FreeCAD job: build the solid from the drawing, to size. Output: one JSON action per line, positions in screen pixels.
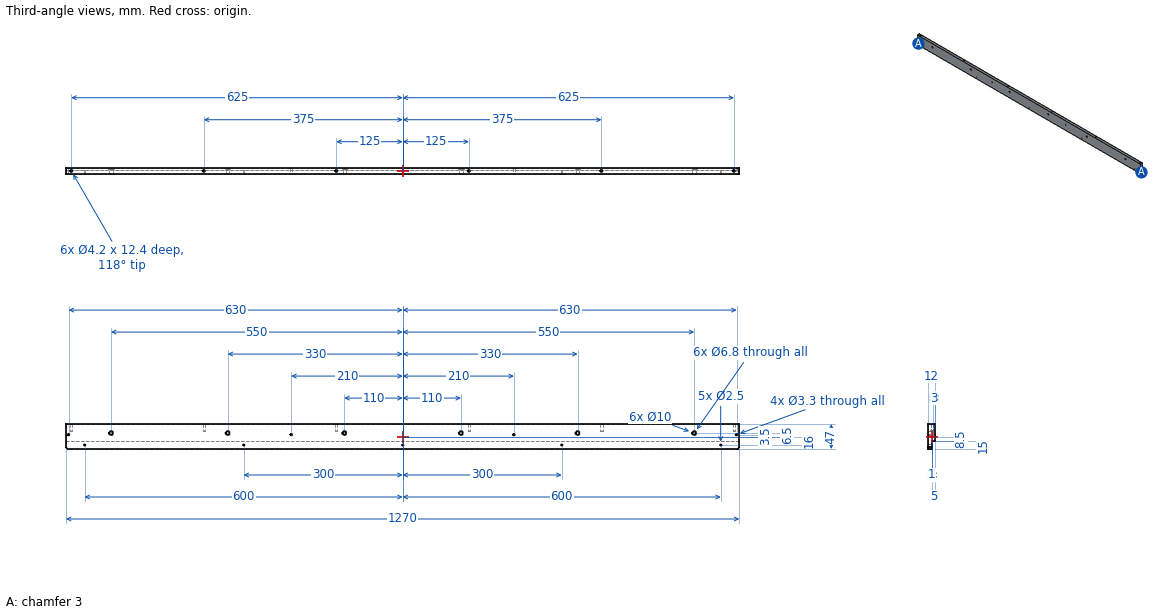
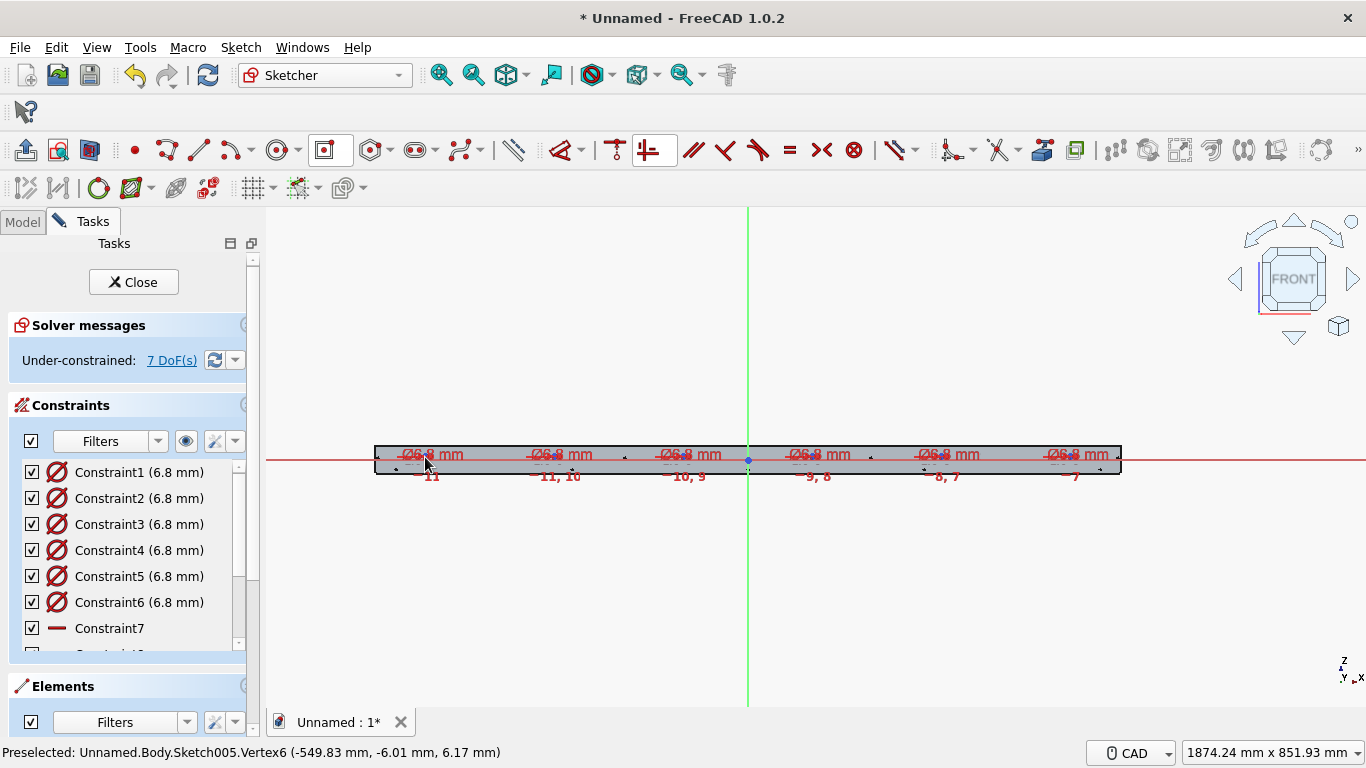
{"action": "key", "text": "d"}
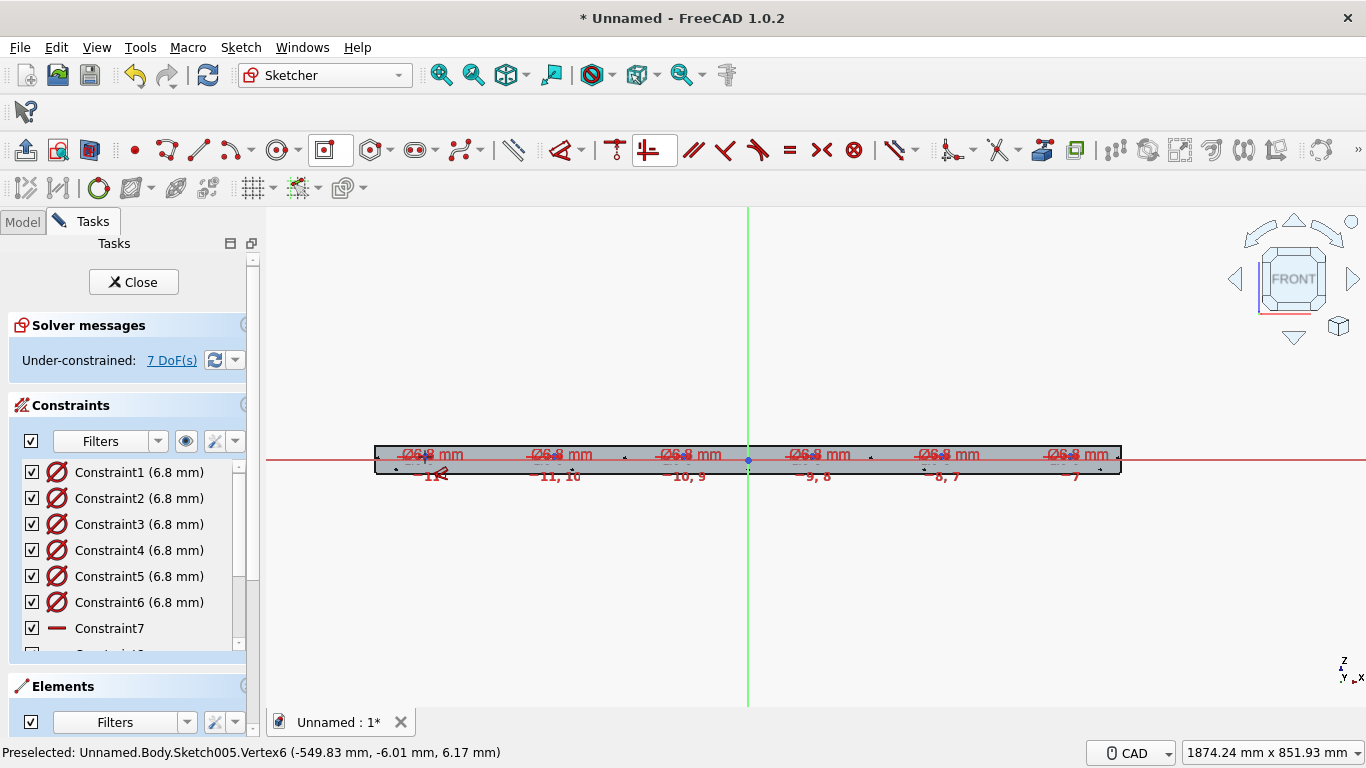
{"action": "left_click", "coordinate": [1071, 457]}
{"action": "left_click", "coordinate": [909, 494]}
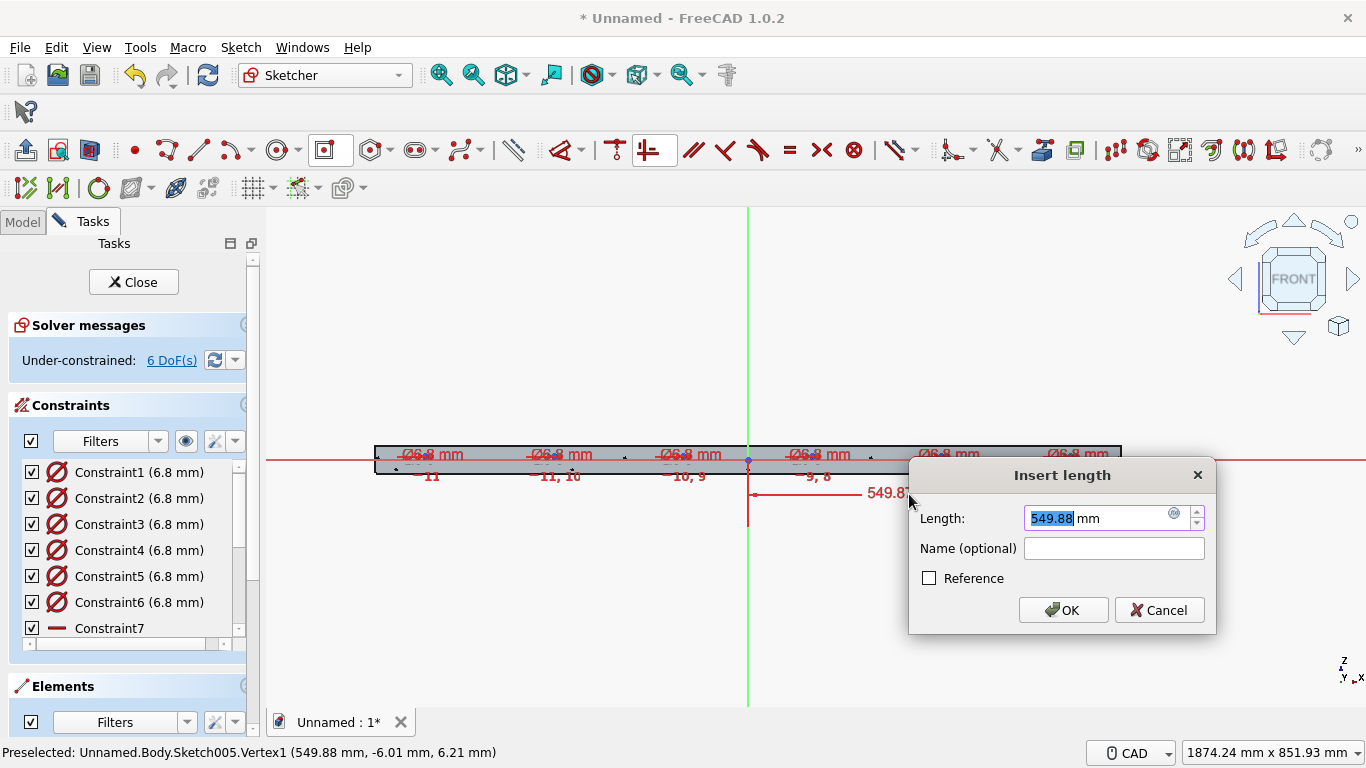
{"action": "type", "text": "550"}
{"action": "key", "text": "Return"}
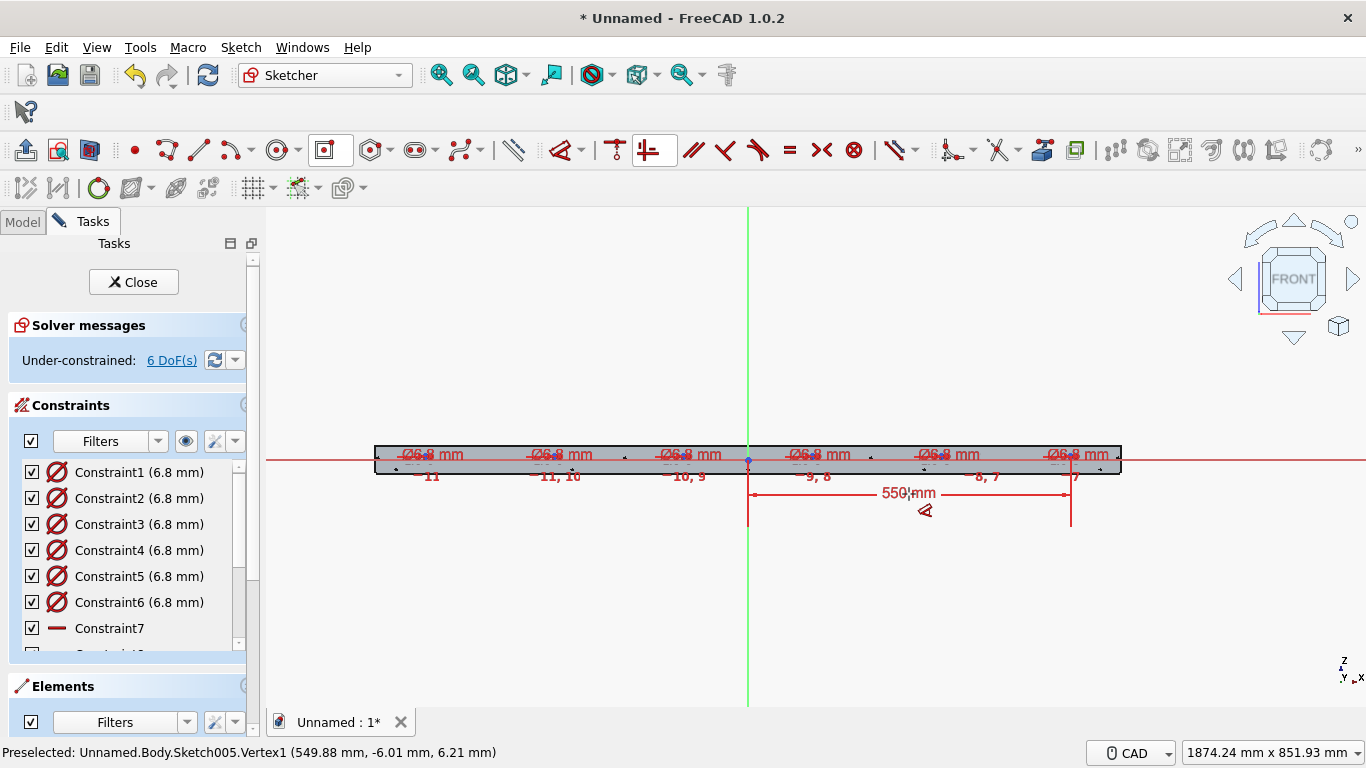
{"action": "scroll", "coordinate": [1071, 457], "scroll_direction": "up", "scroll_amount": 12}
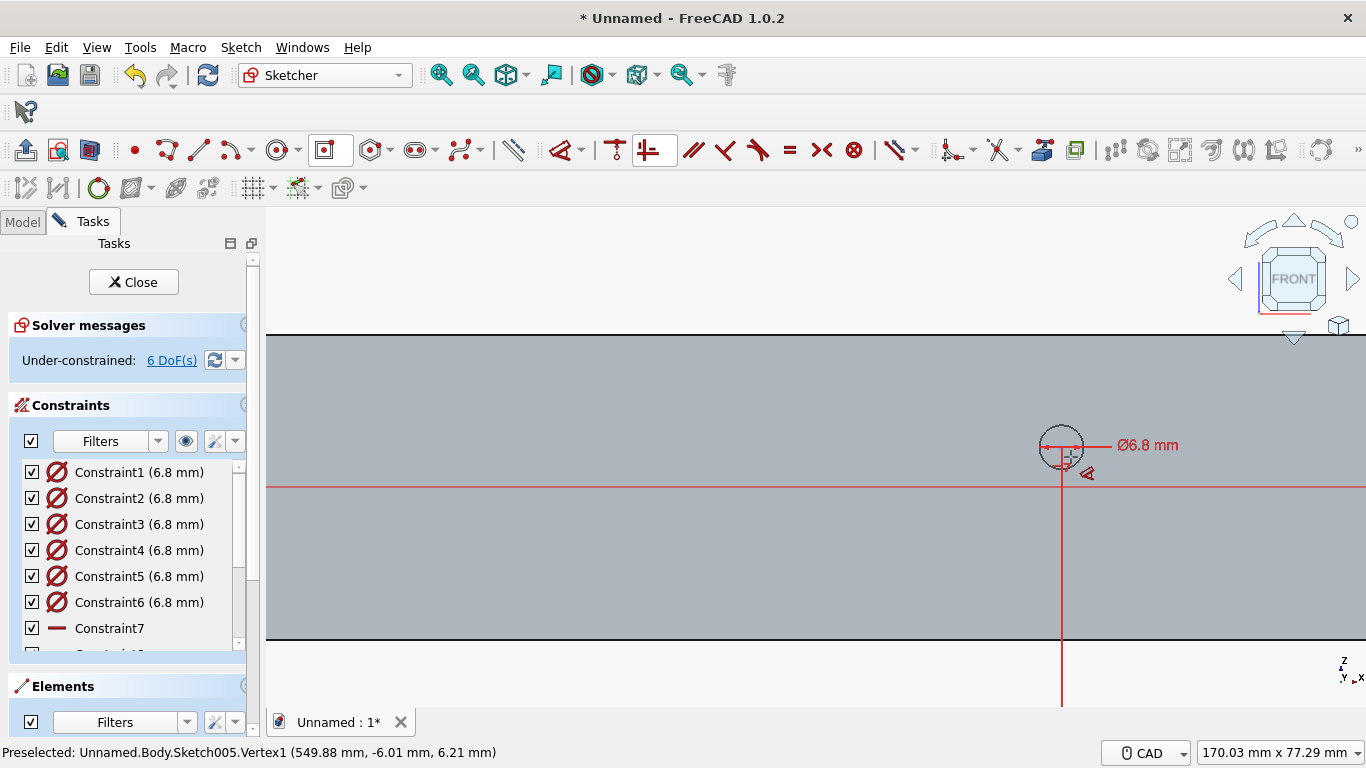
{"action": "left_click", "coordinate": [1062, 447]}
{"action": "left_click", "coordinate": [1096, 467]}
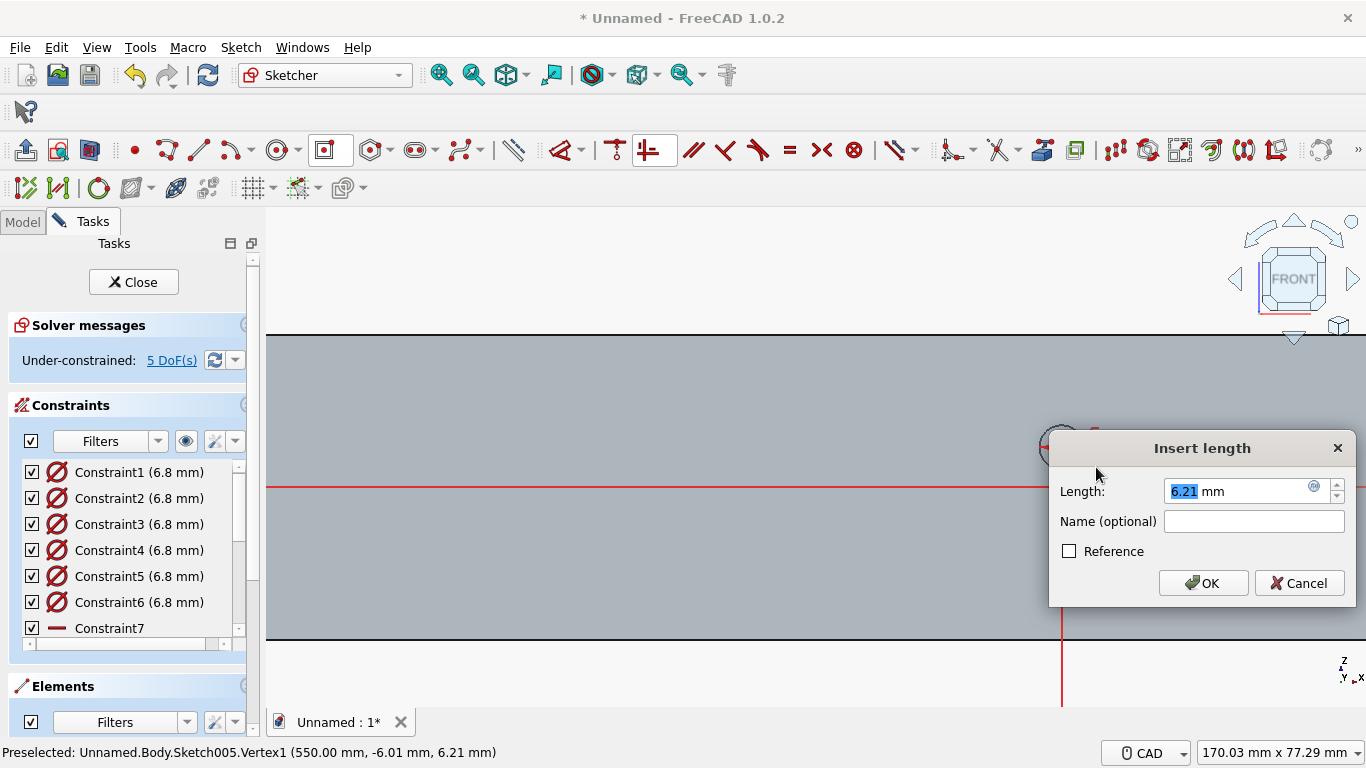
{"action": "type", "text": "6.5"}
{"action": "key", "text": "Return"}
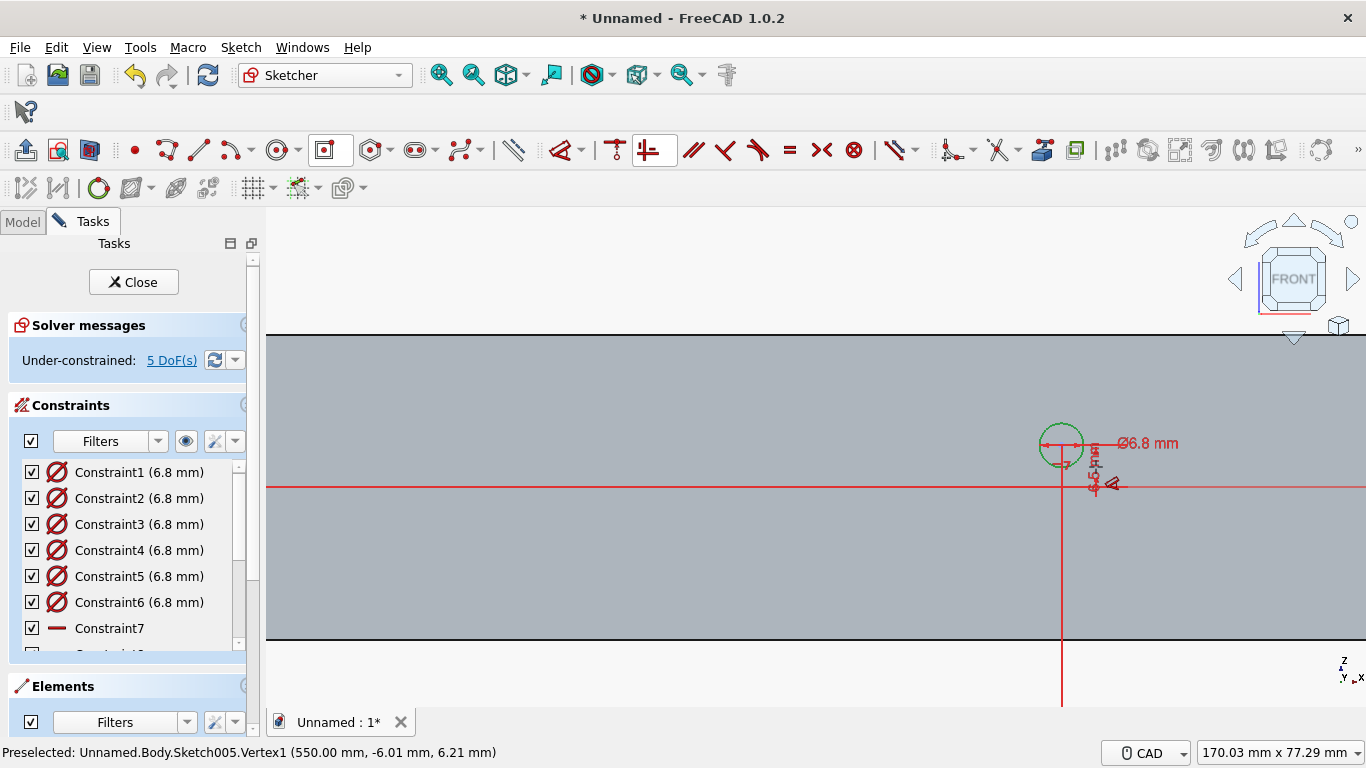
{"action": "scroll", "coordinate": [1071, 457], "scroll_direction": "down", "scroll_amount": 12}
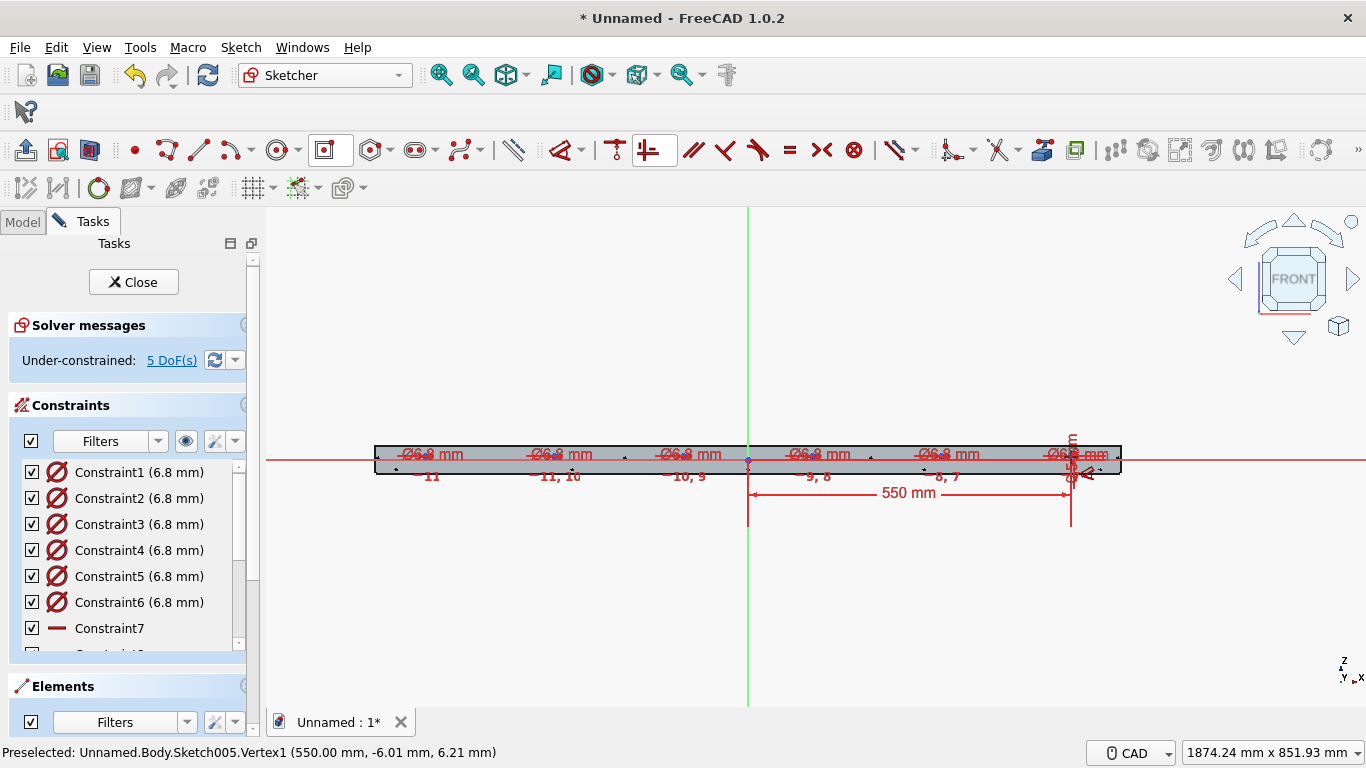
{"action": "left_click", "coordinate": [942, 456]}
{"action": "left_click", "coordinate": [800, 494]}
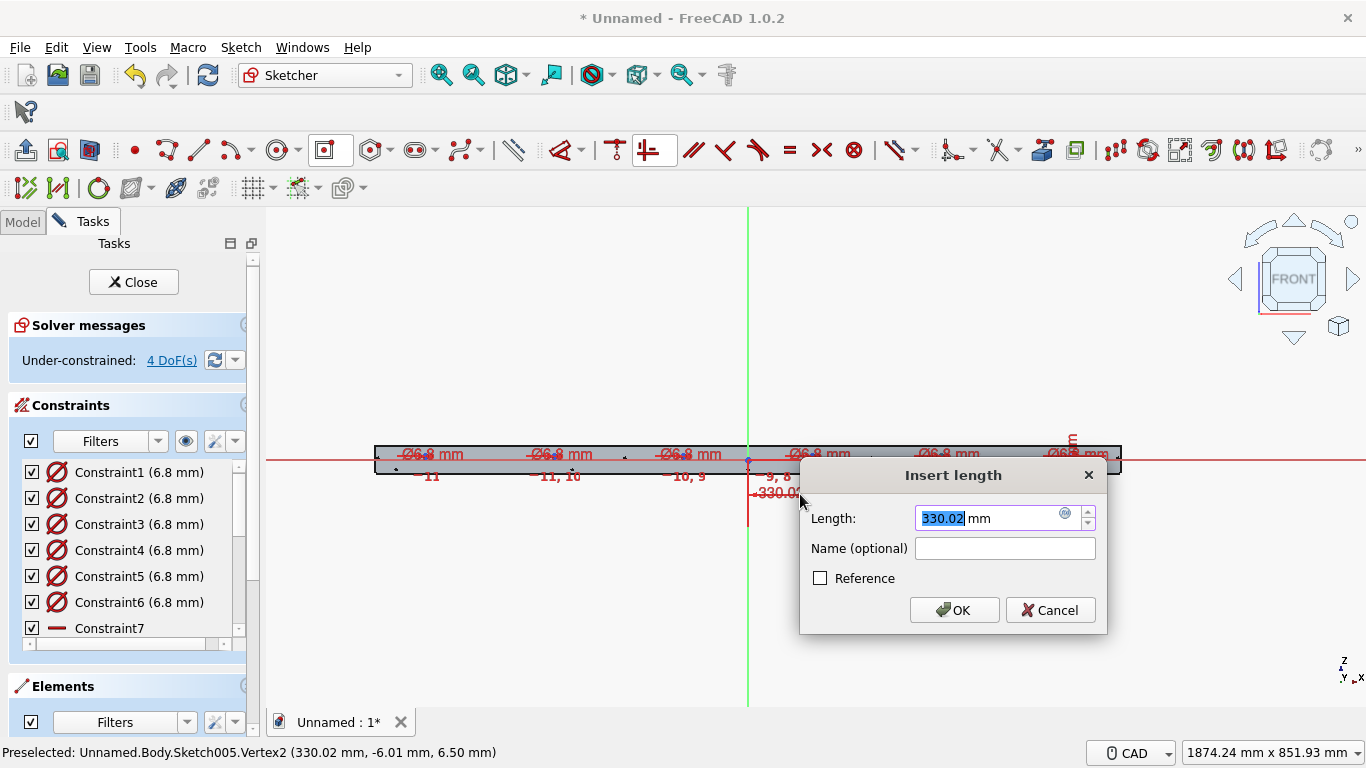
{"action": "type", "text": "330"}
{"action": "key", "text": "Return"}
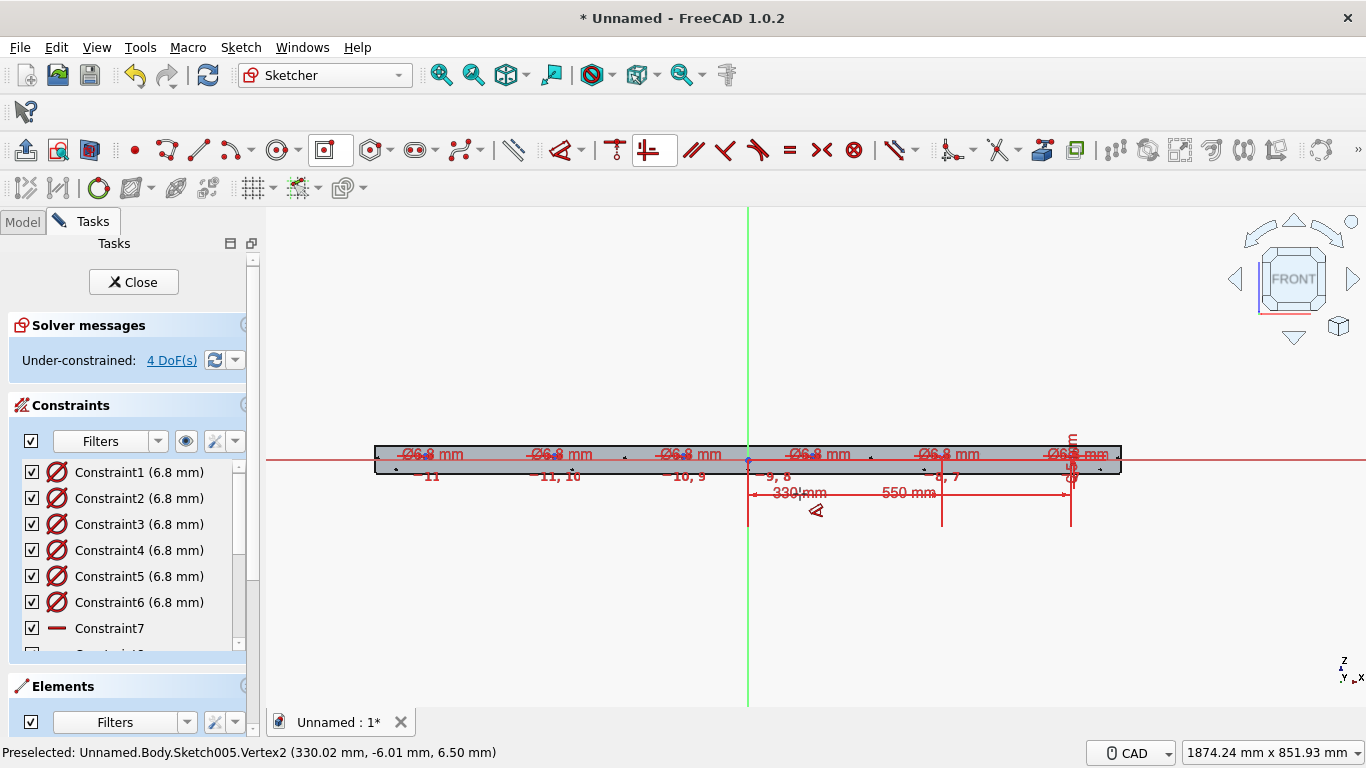
{"action": "left_click", "coordinate": [813, 456]}
{"action": "left_click", "coordinate": [780, 422]}